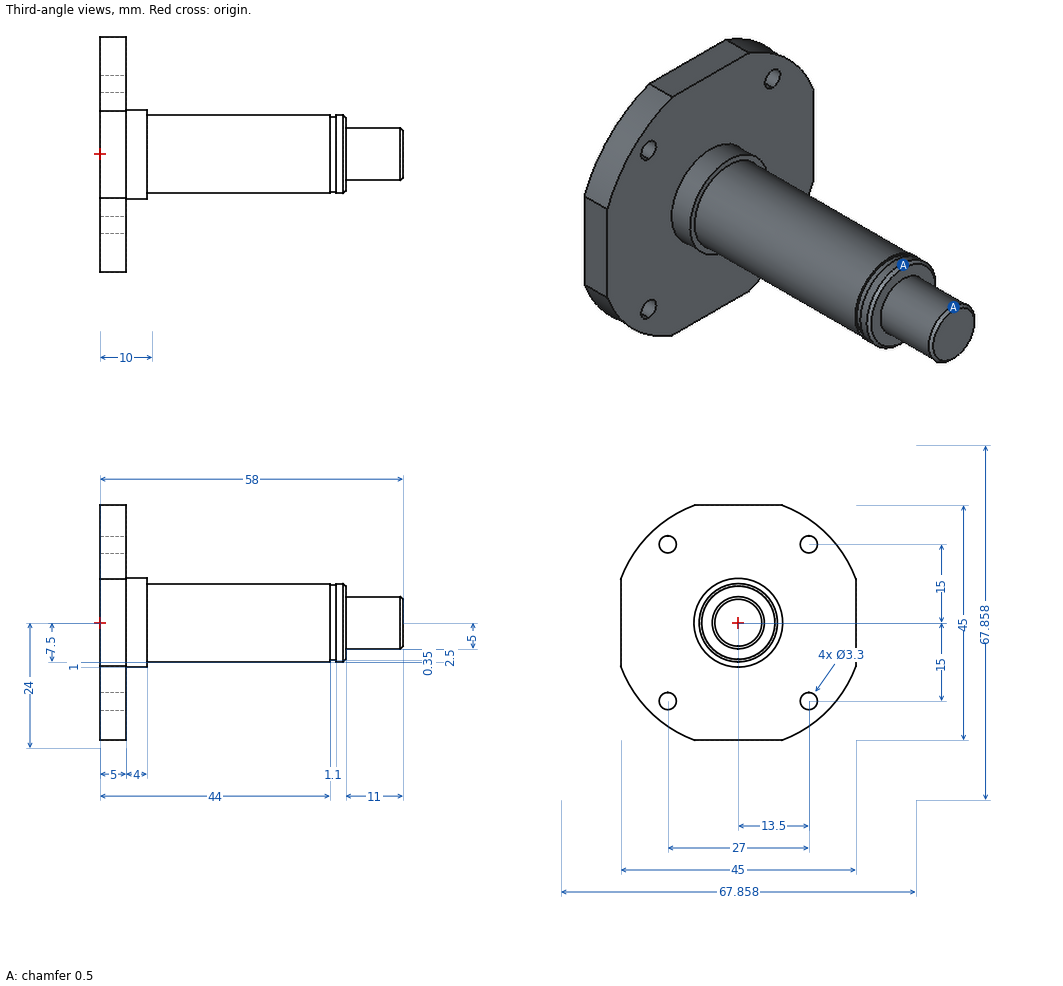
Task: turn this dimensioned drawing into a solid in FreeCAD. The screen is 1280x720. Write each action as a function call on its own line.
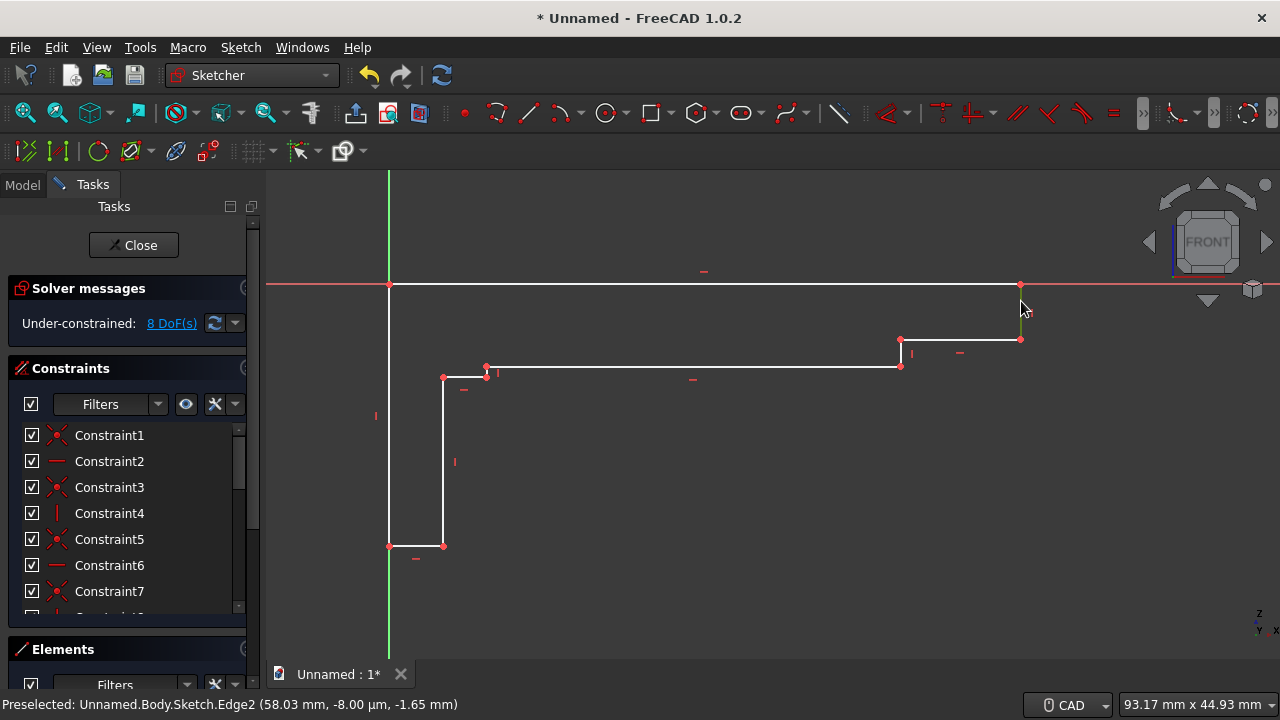
click(910, 114)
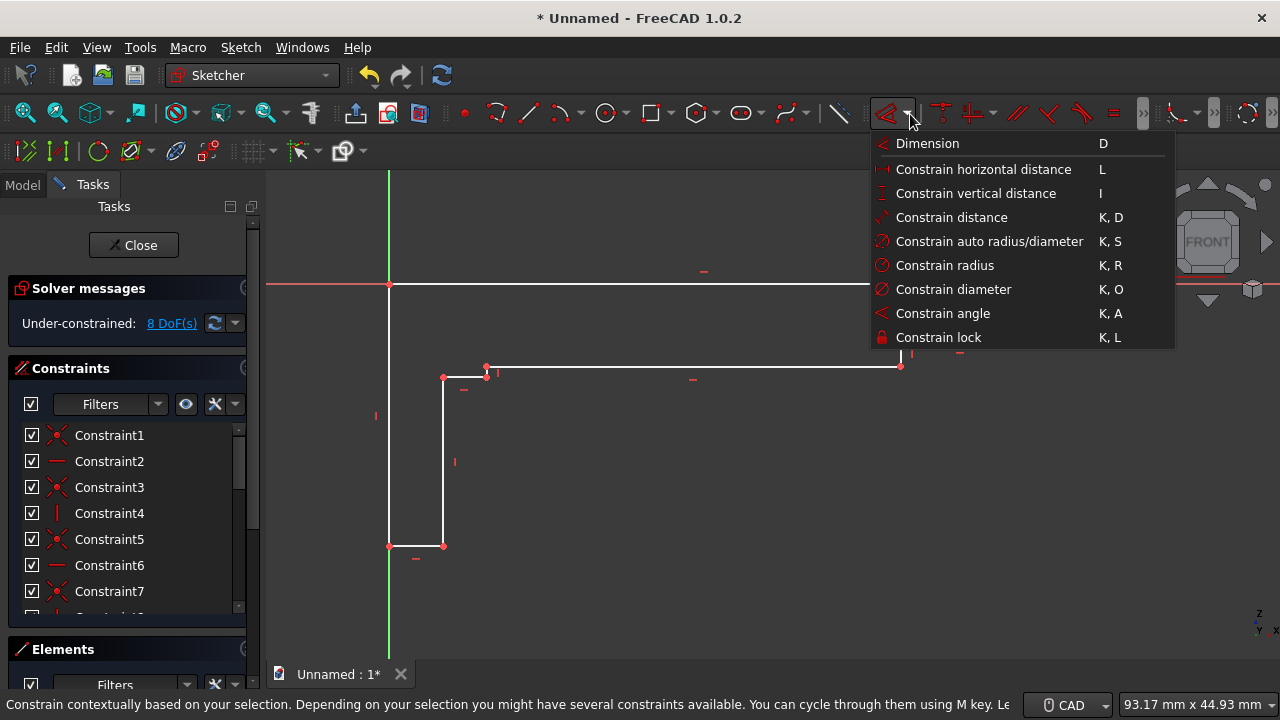
click(1023, 193)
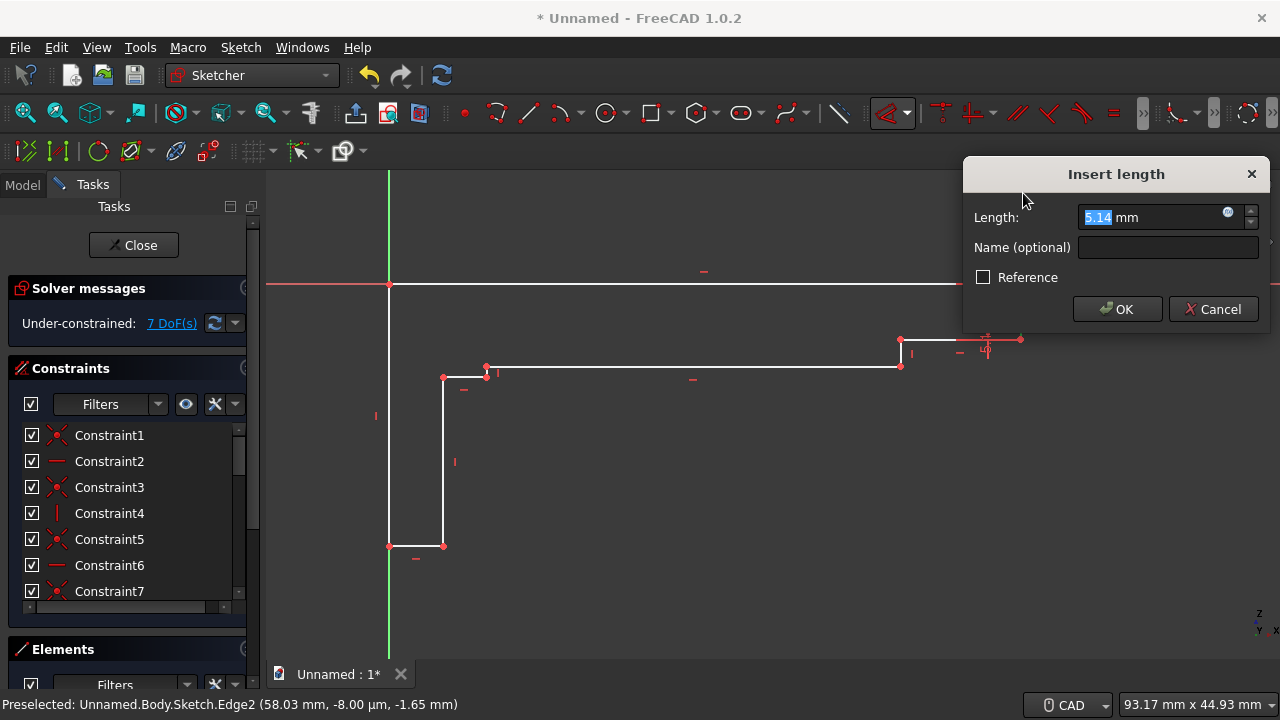
text(5)
key(Return)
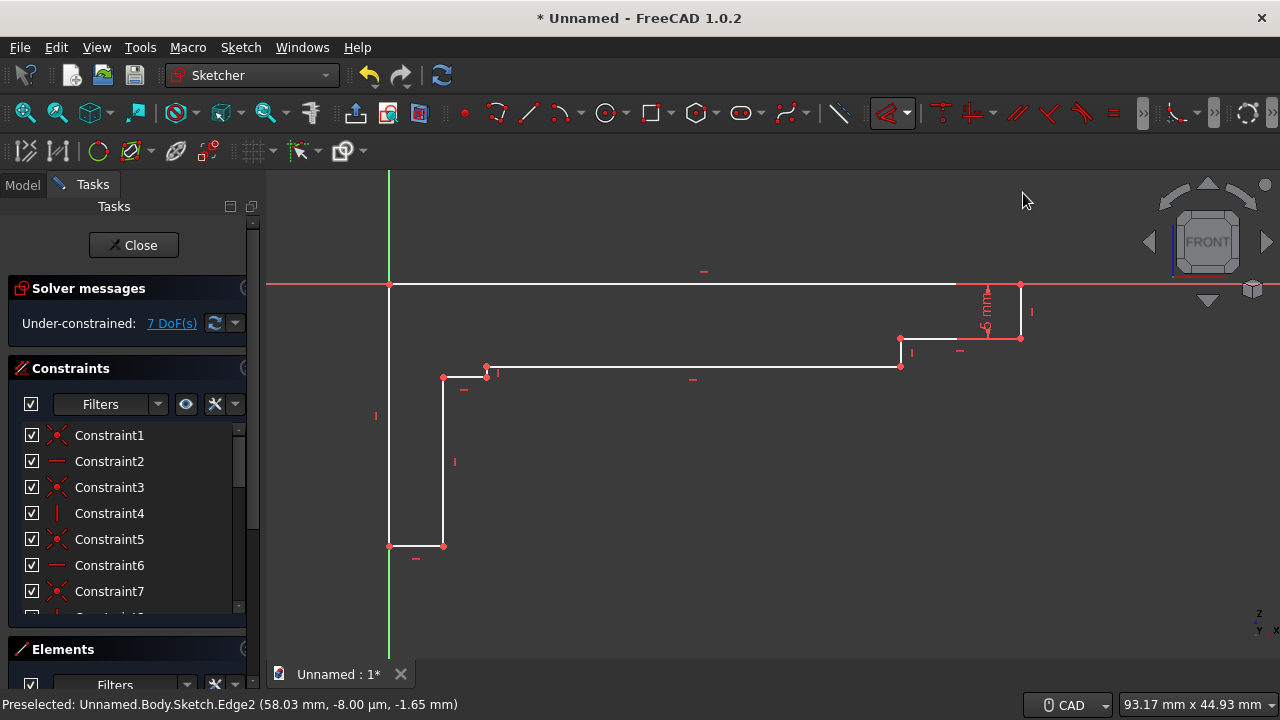
scroll(487, 372, up, 7)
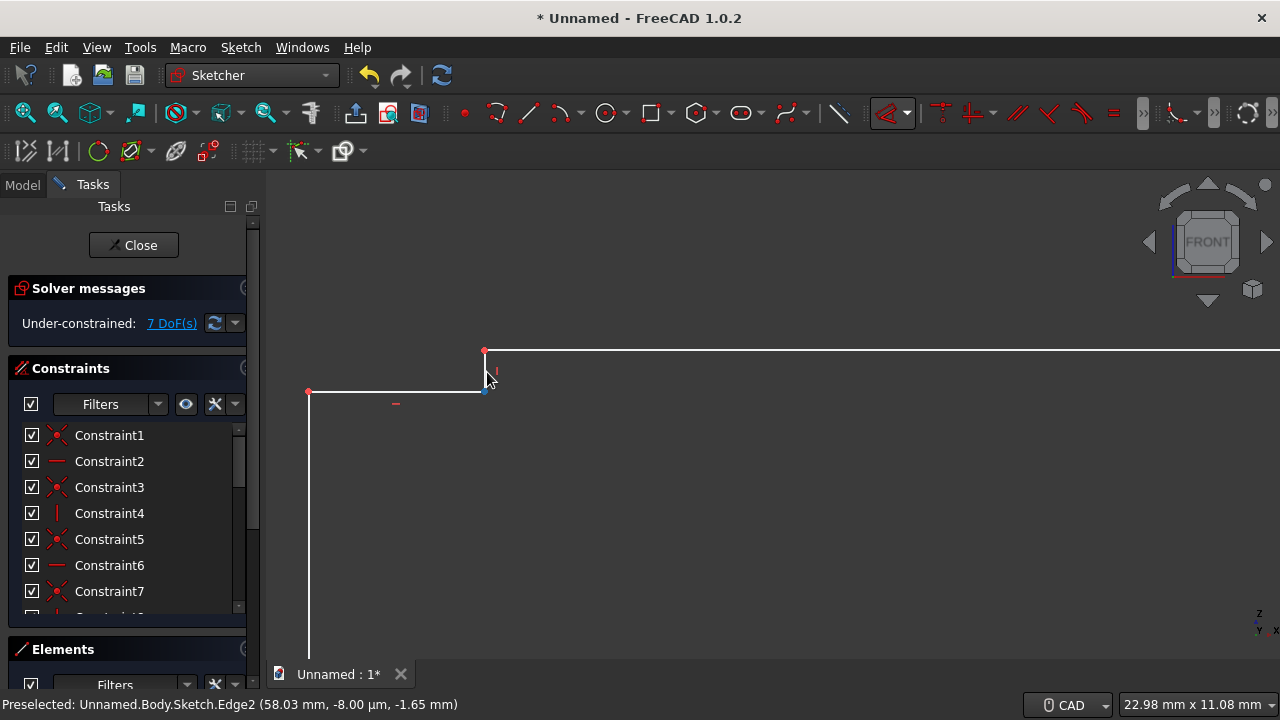
click(485, 371)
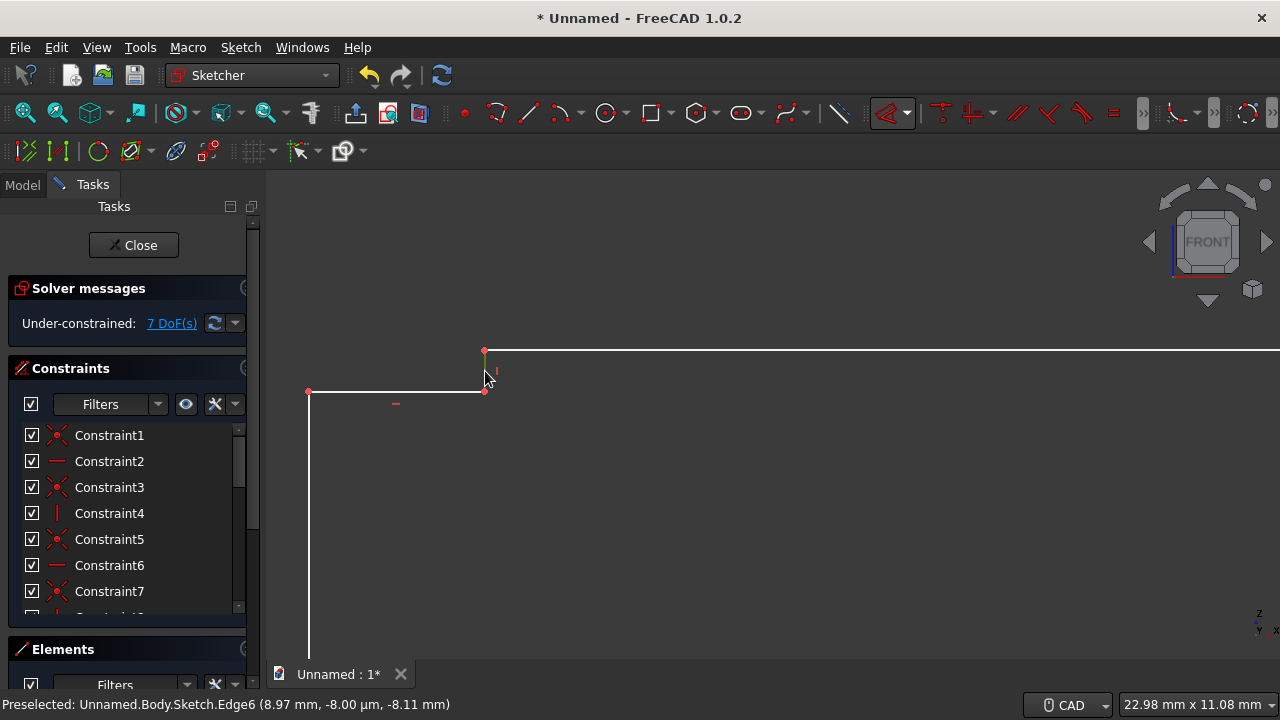
click(910, 114)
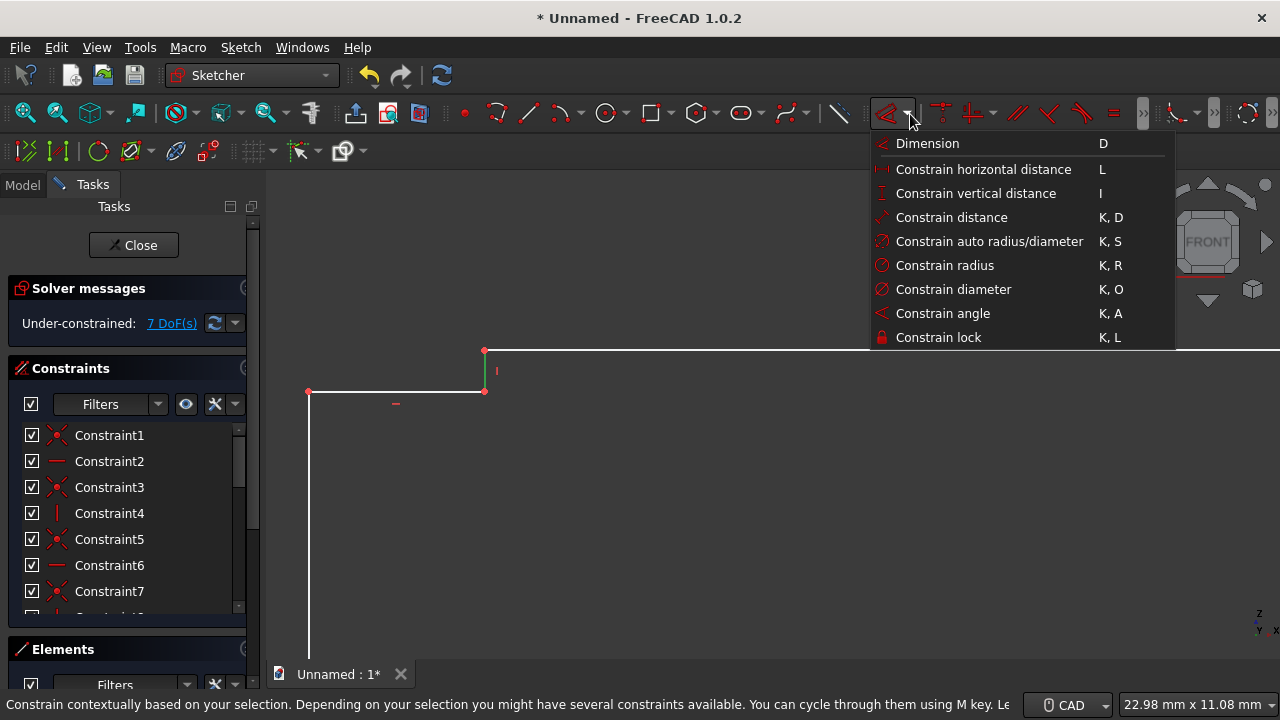
click(1023, 193)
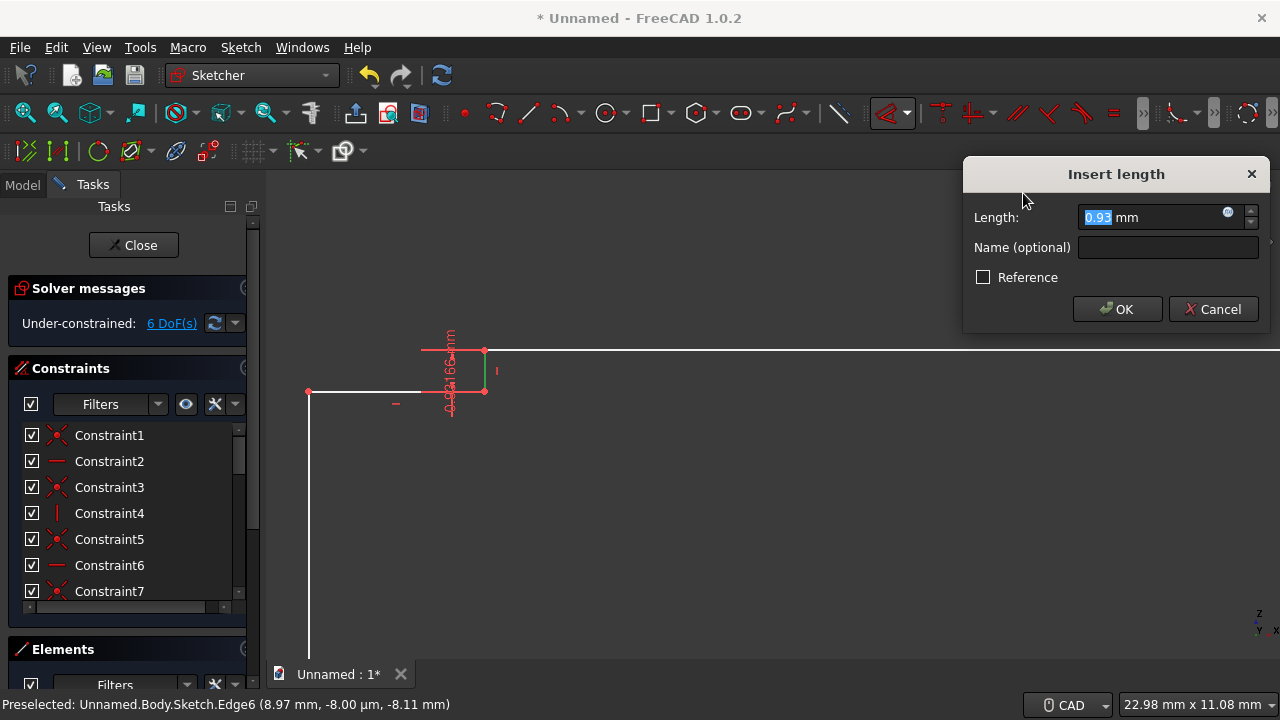
text(1)
key(Return)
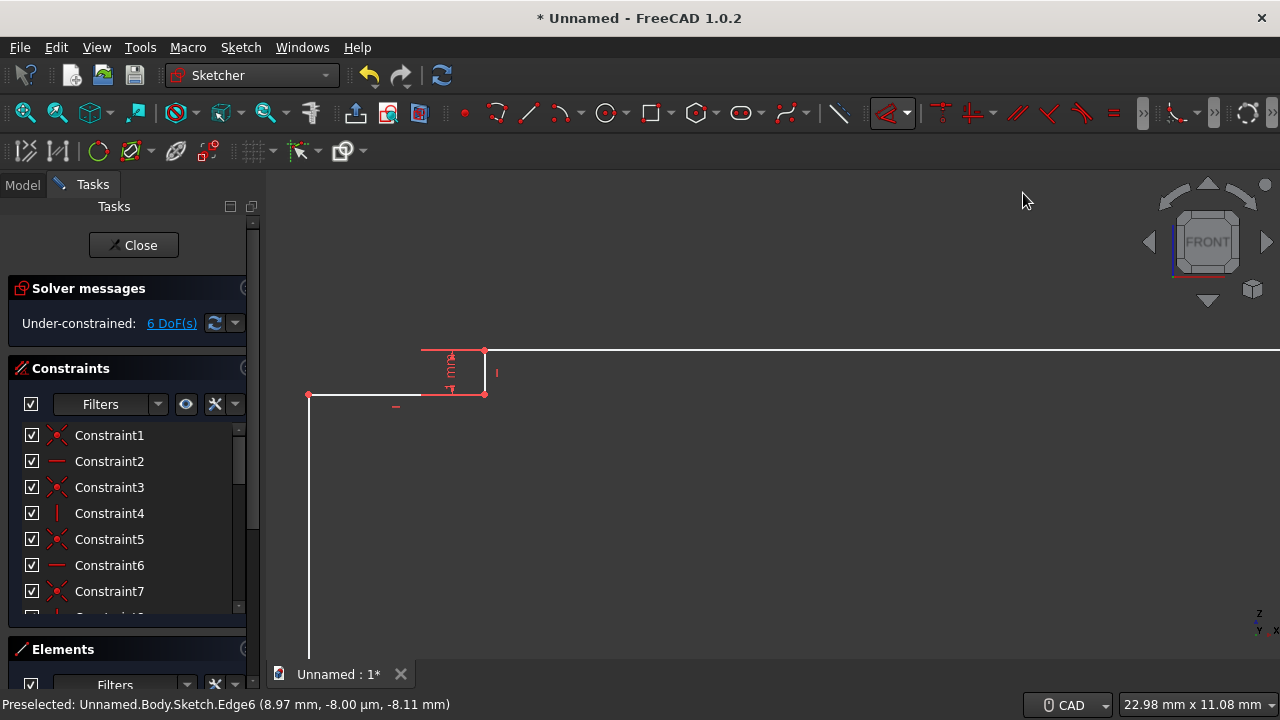
scroll(487, 372, down, 7)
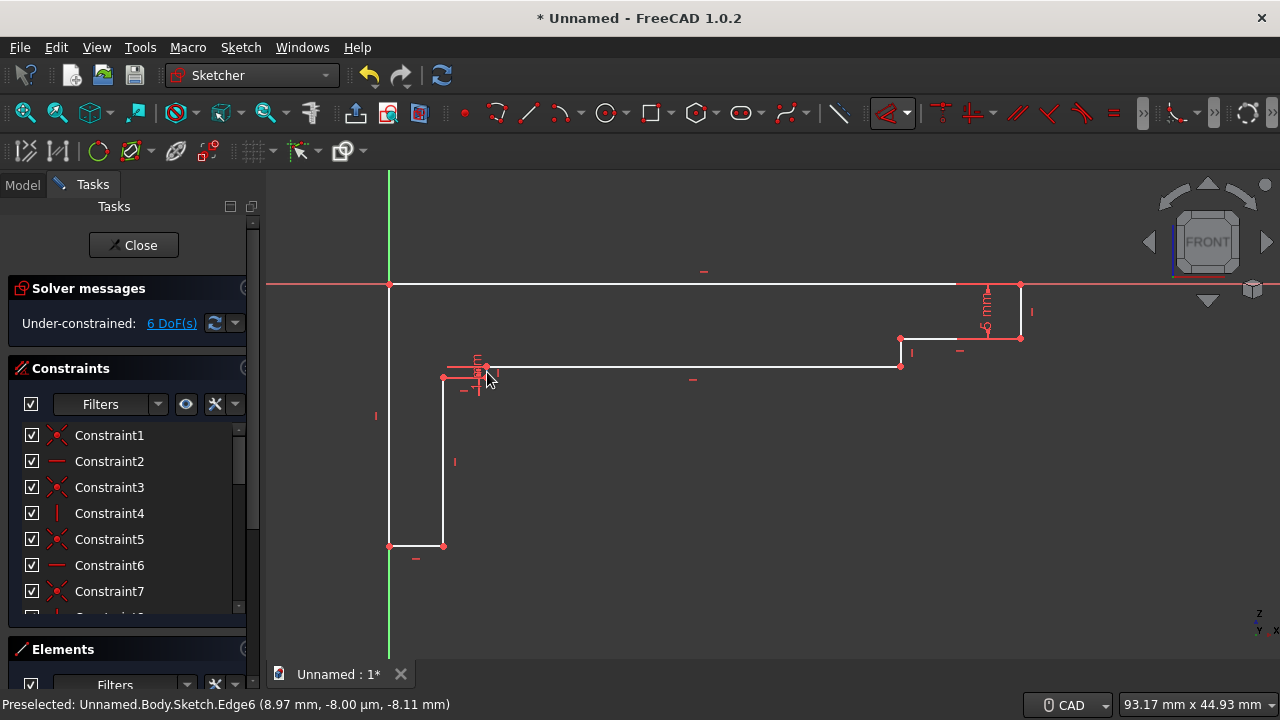
click(456, 378)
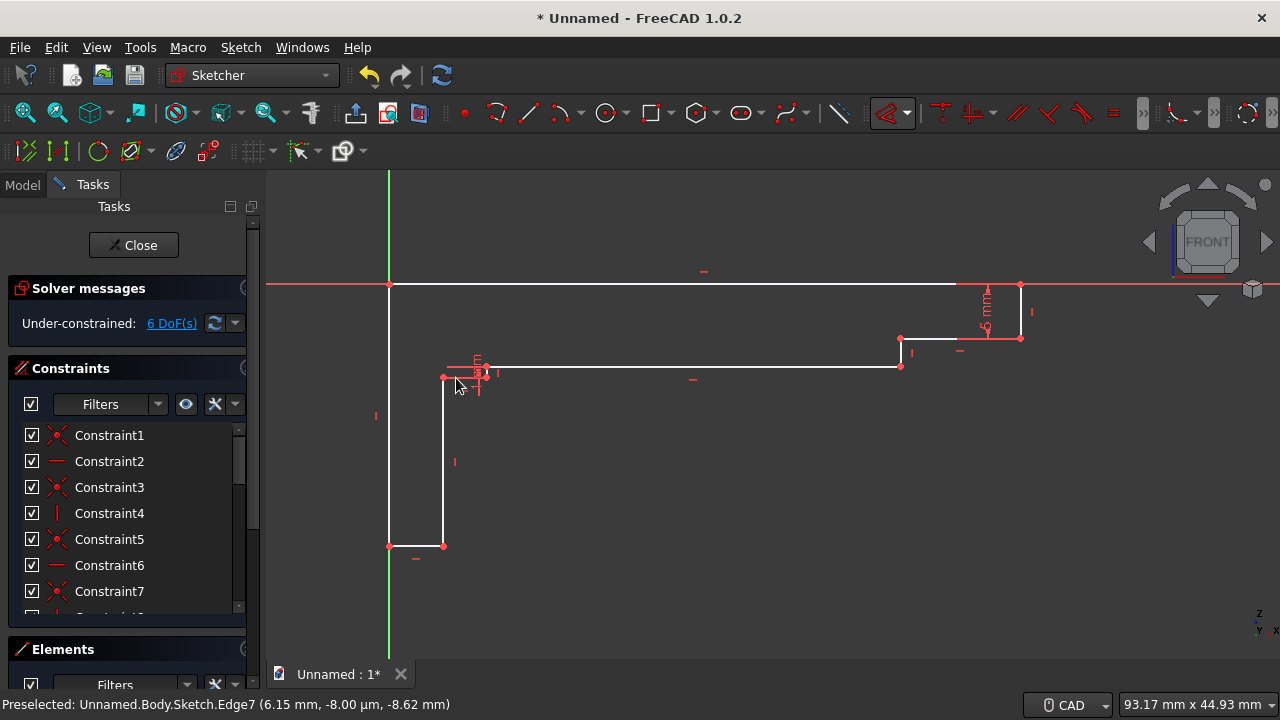
click(910, 114)